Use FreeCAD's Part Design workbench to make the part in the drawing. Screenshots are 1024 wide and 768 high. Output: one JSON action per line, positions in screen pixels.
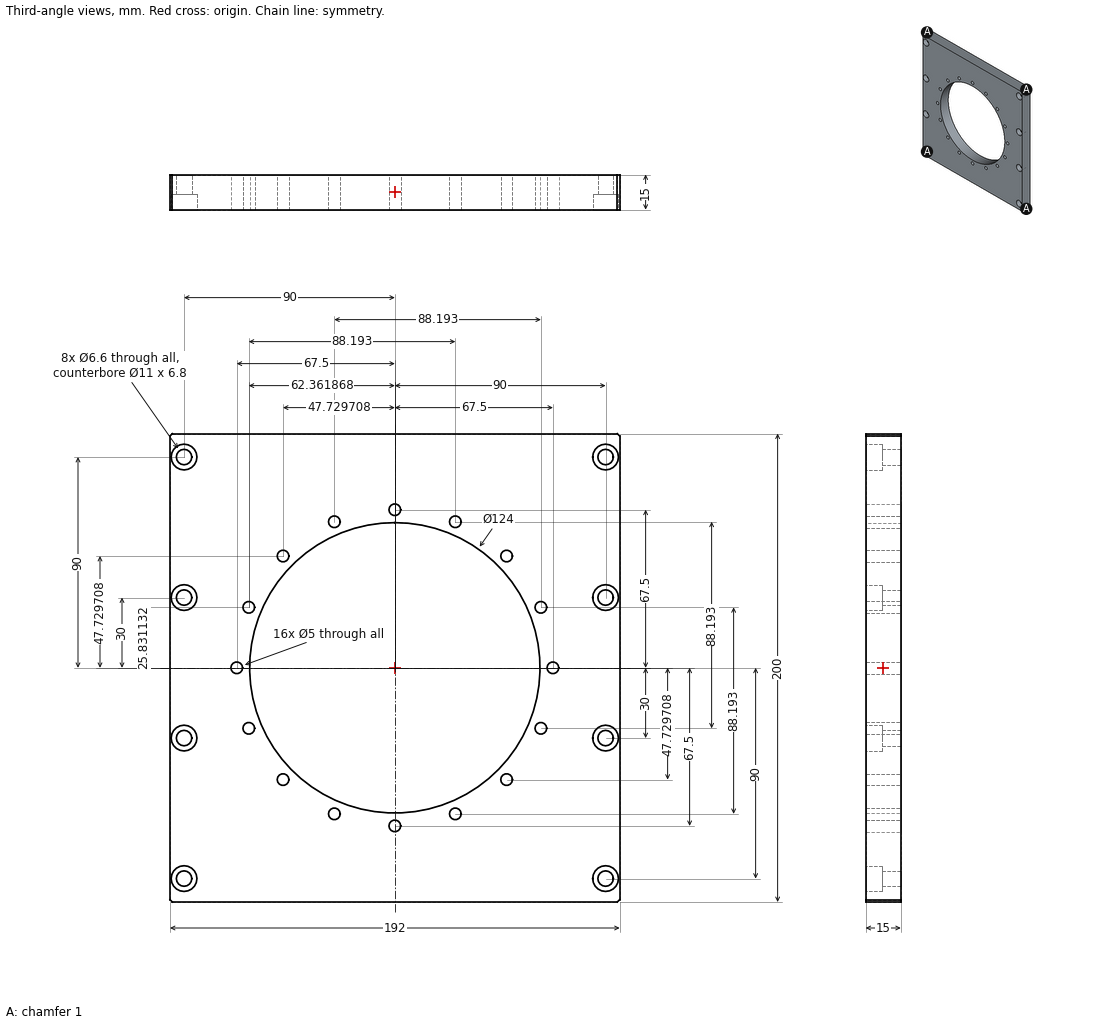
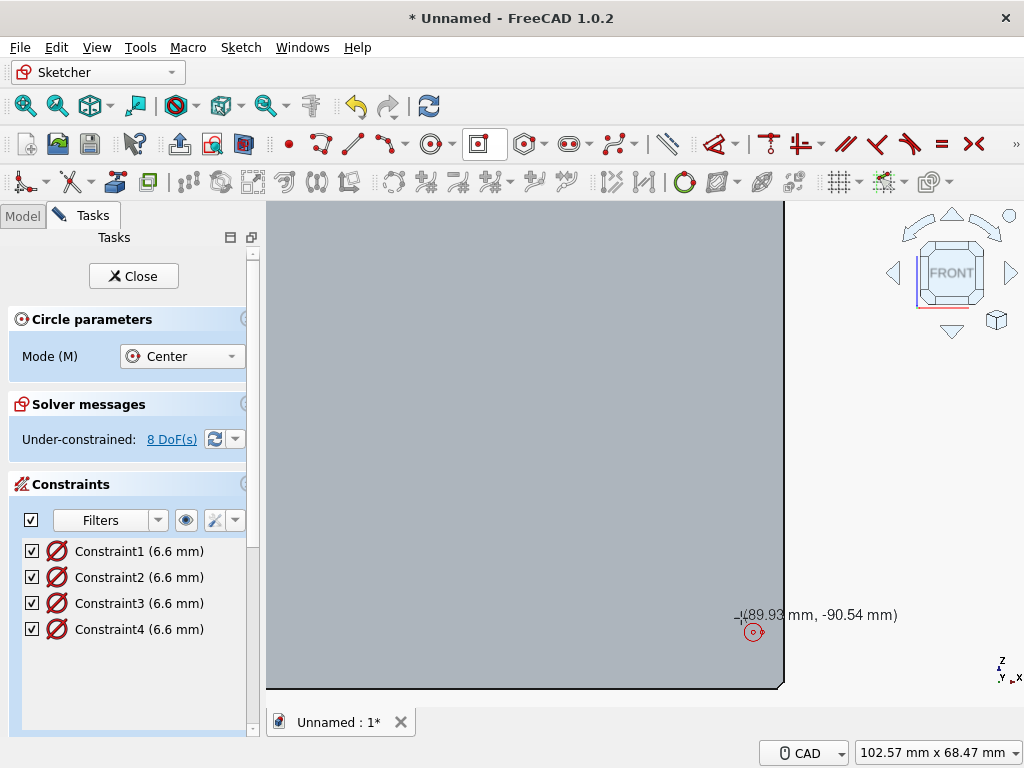
{"action": "scroll", "coordinate": [741, 619], "scroll_direction": "down", "scroll_amount": 7}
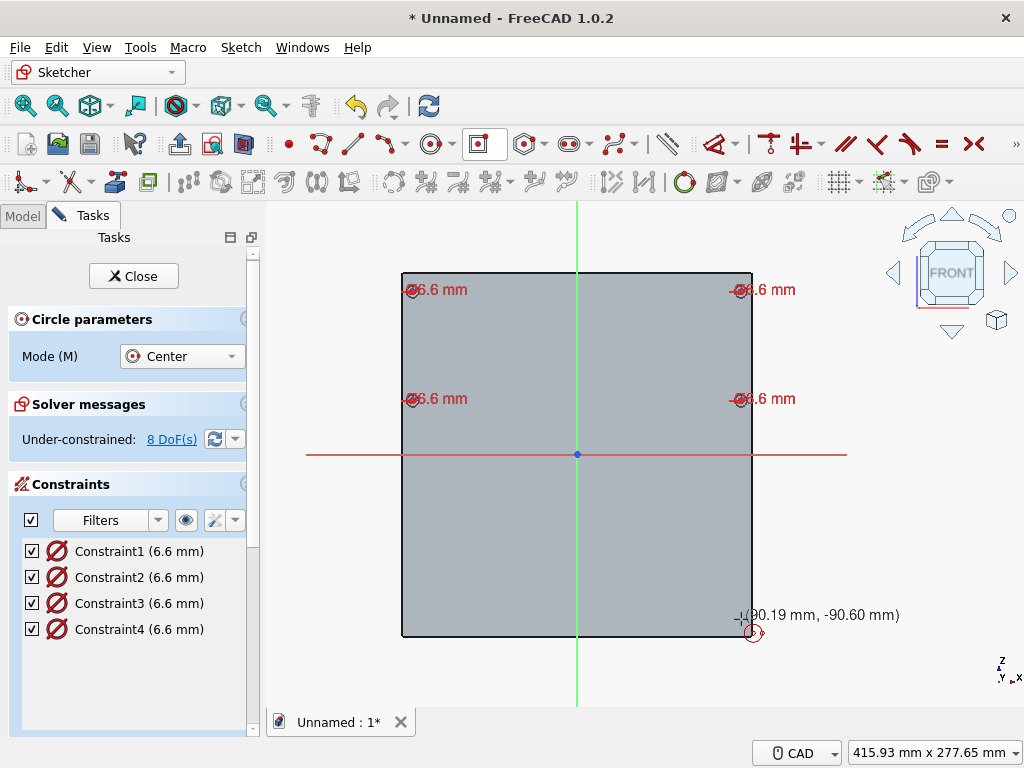
{"action": "left_click", "coordinate": [741, 619]}
{"action": "mouse_move", "coordinate": [745, 615]}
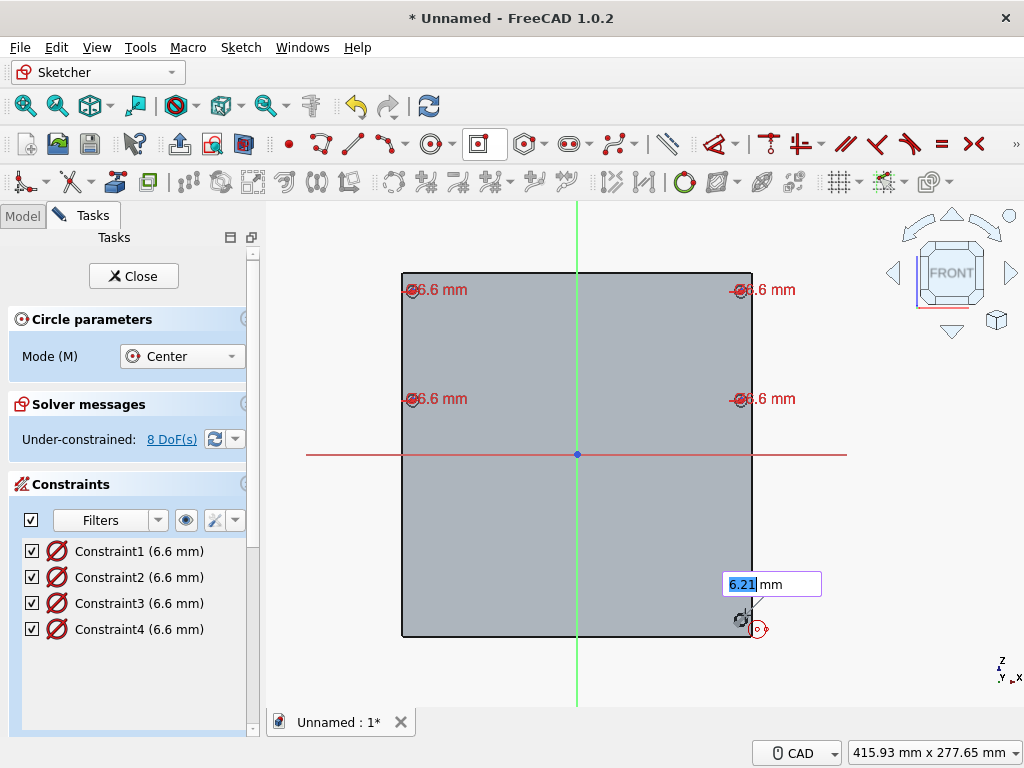
{"action": "type", "text": "6.6"}
{"action": "key", "text": "Return"}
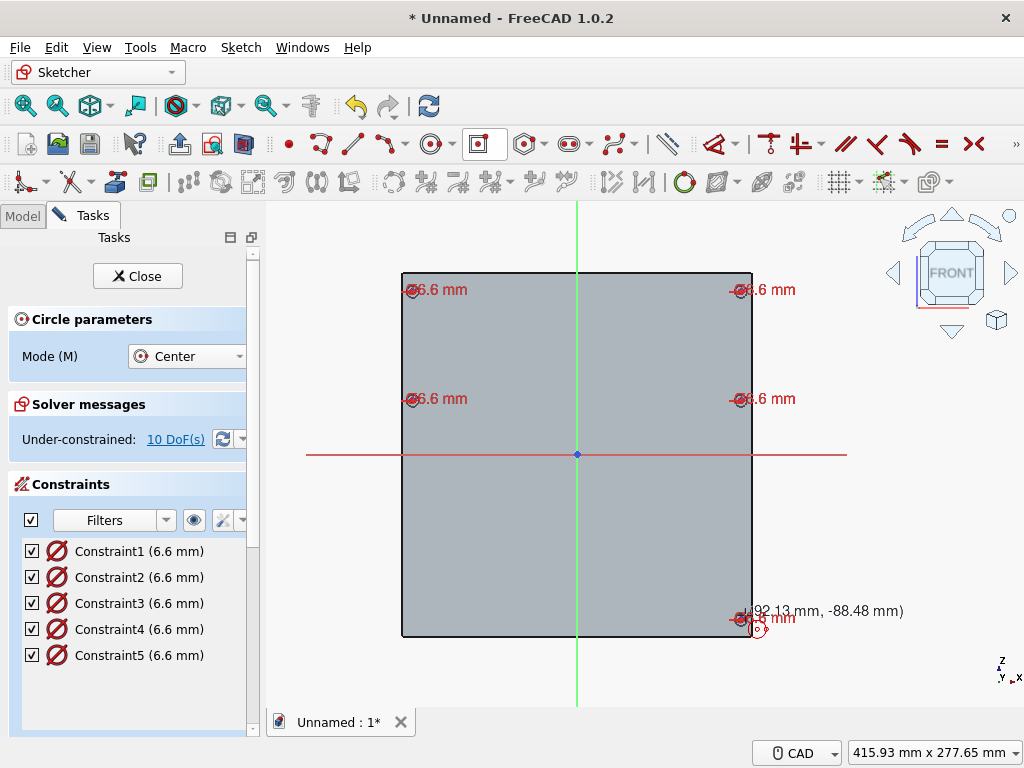
{"action": "scroll", "coordinate": [741, 509], "scroll_direction": "up", "scroll_amount": 7}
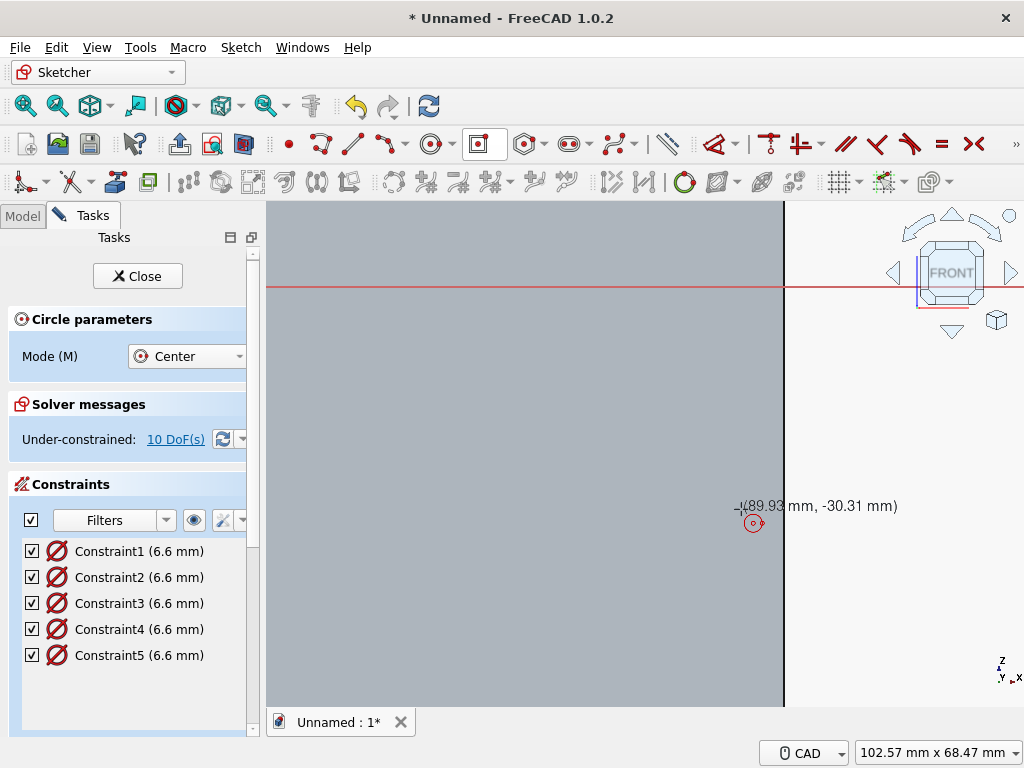
{"action": "scroll", "coordinate": [741, 509], "scroll_direction": "down", "scroll_amount": 7}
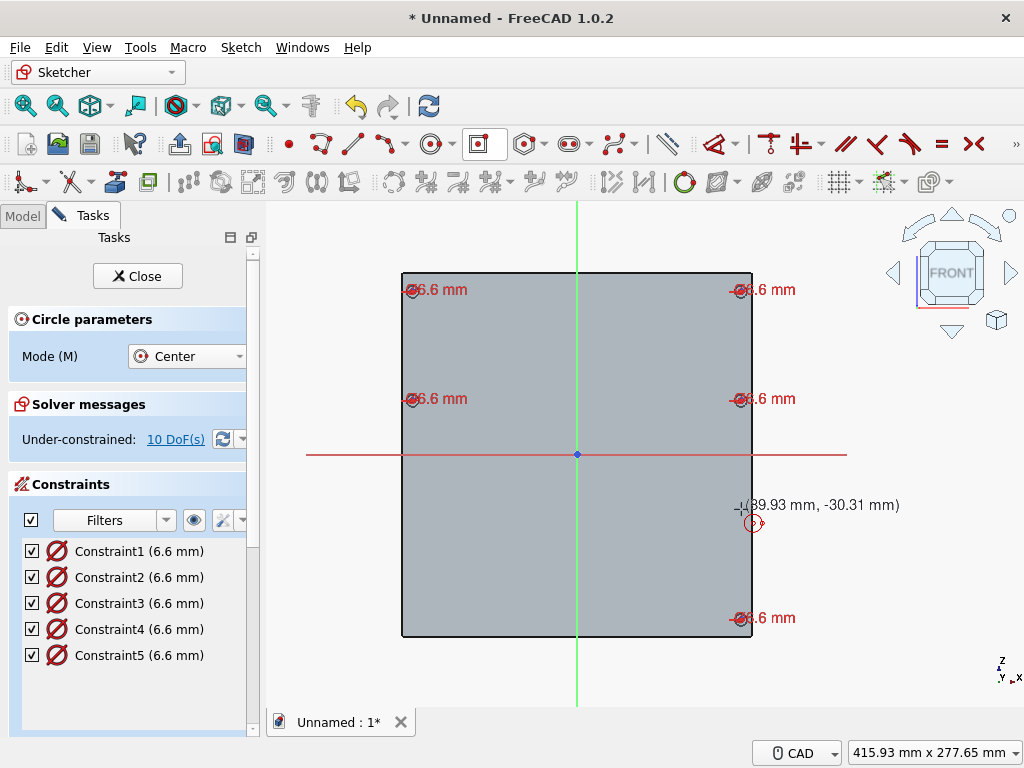
{"action": "left_click", "coordinate": [741, 509]}
{"action": "mouse_move", "coordinate": [745, 505]}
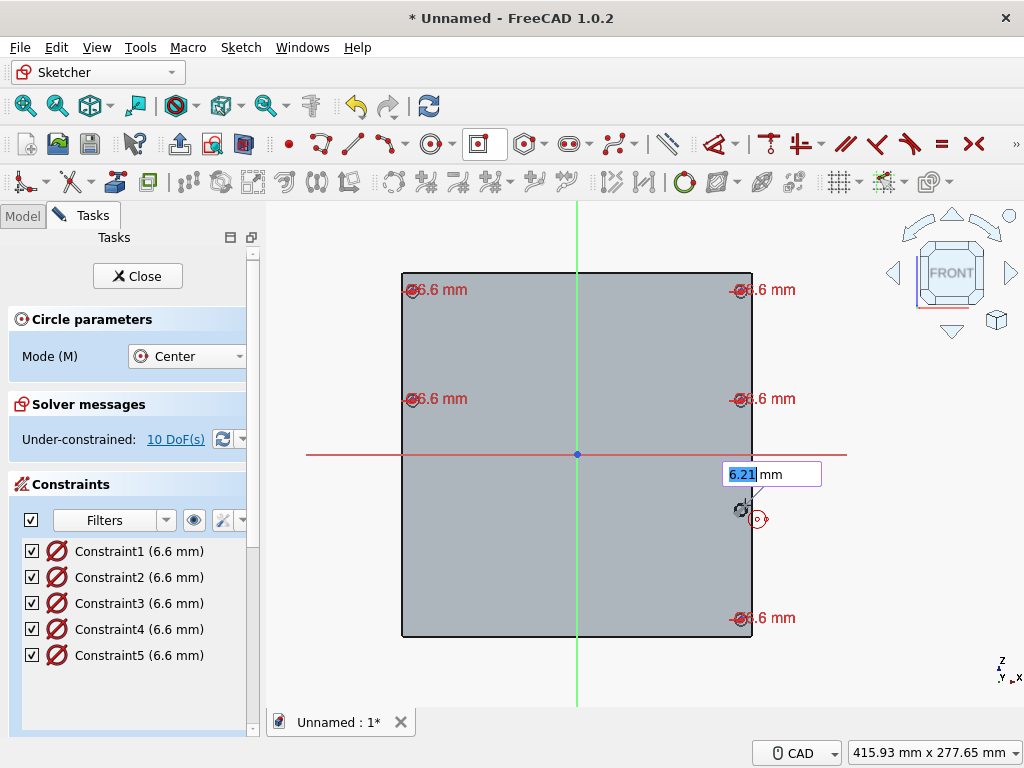
{"action": "type", "text": "6.6"}
{"action": "key", "text": "Return"}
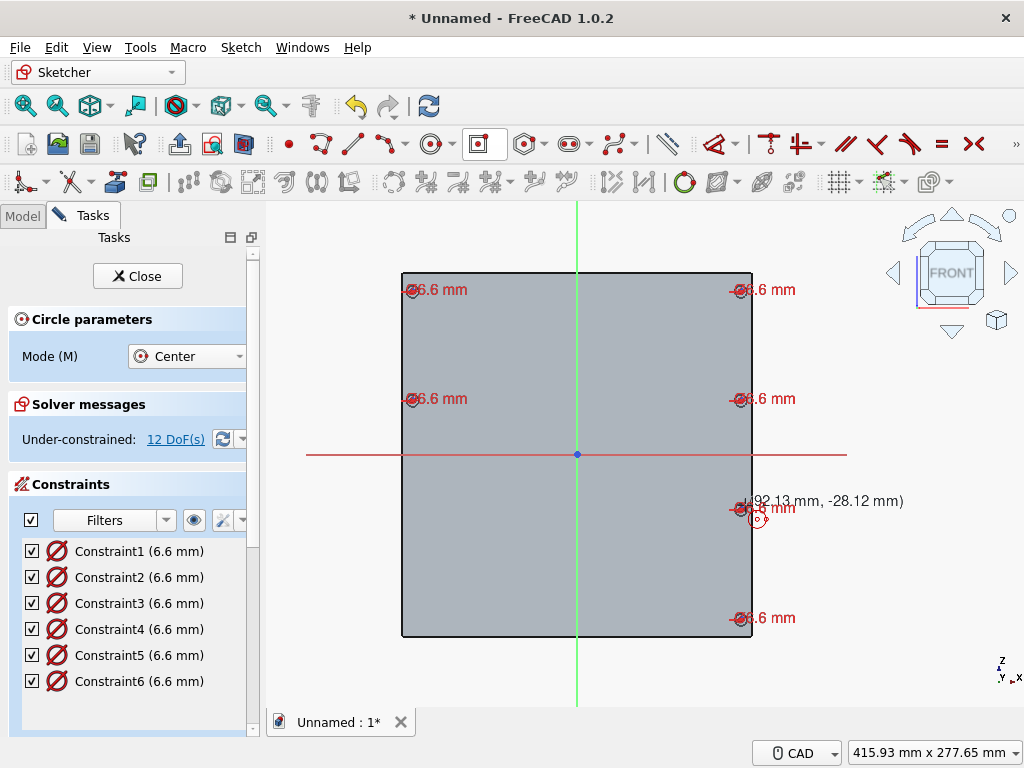
{"action": "scroll", "coordinate": [413, 509], "scroll_direction": "up", "scroll_amount": 7}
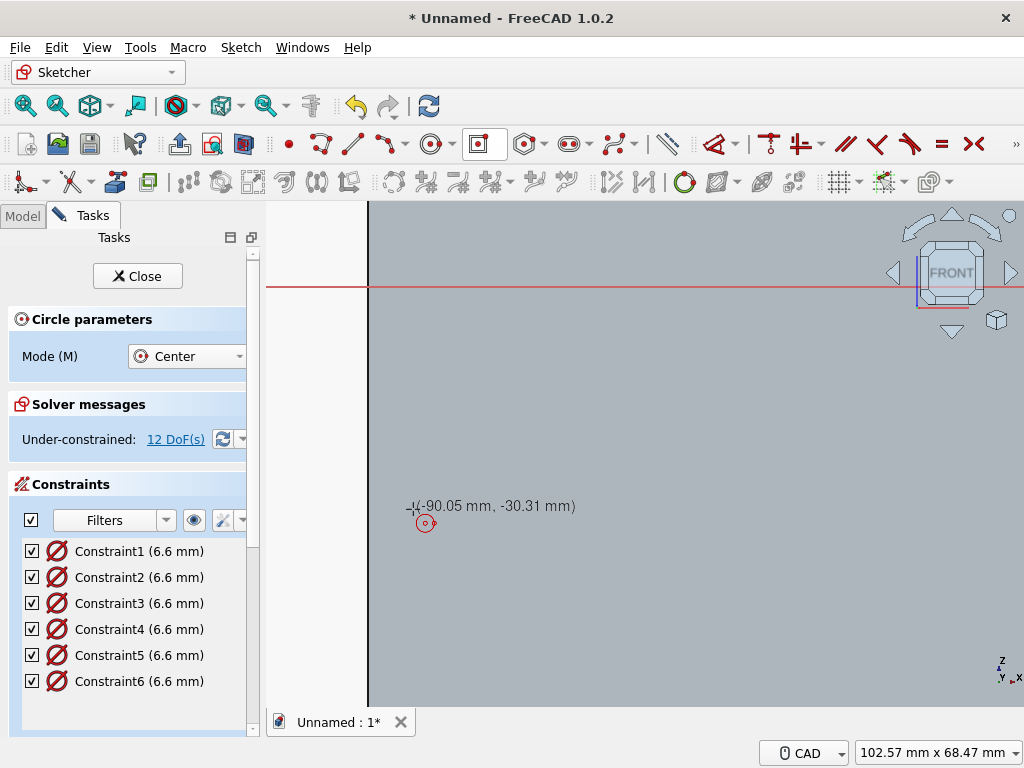
{"action": "scroll", "coordinate": [412, 509], "scroll_direction": "down", "scroll_amount": 7}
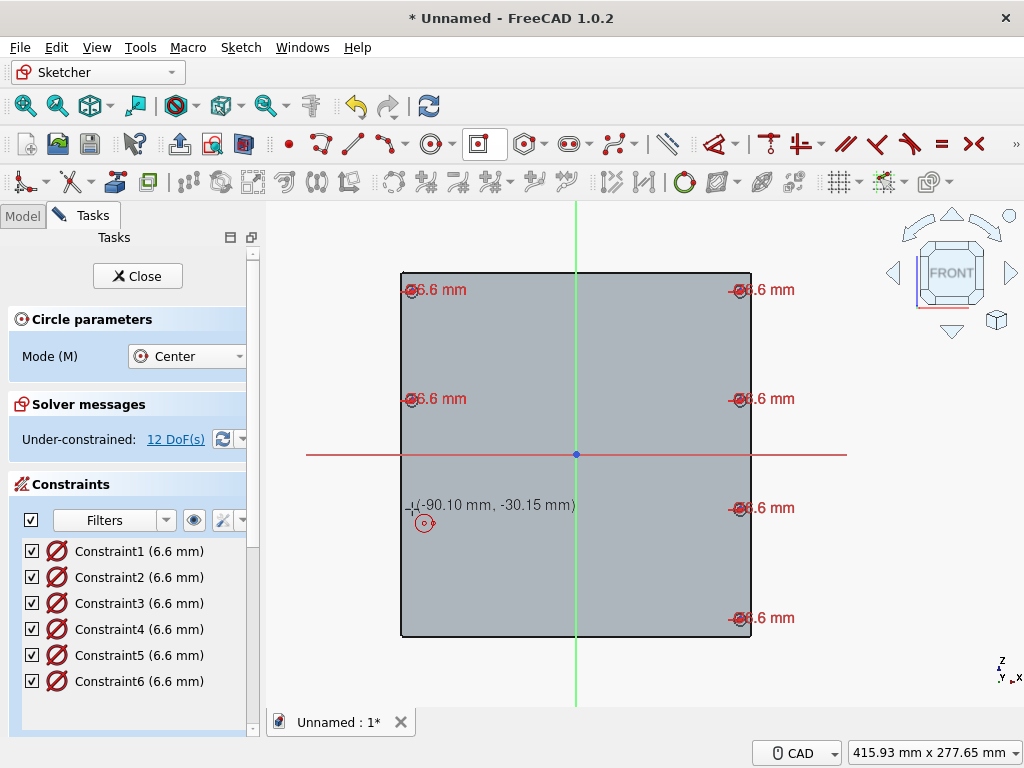
{"action": "left_click", "coordinate": [412, 509]}
{"action": "mouse_move", "coordinate": [417, 505]}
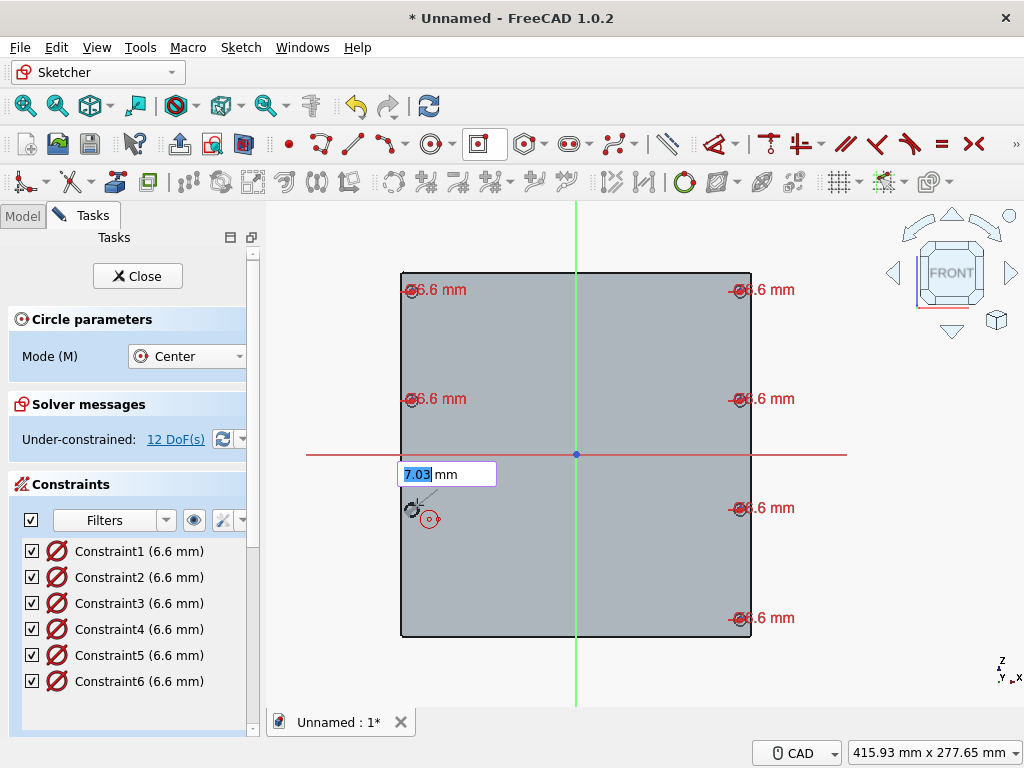
{"action": "type", "text": "6.6"}
{"action": "key", "text": "Return"}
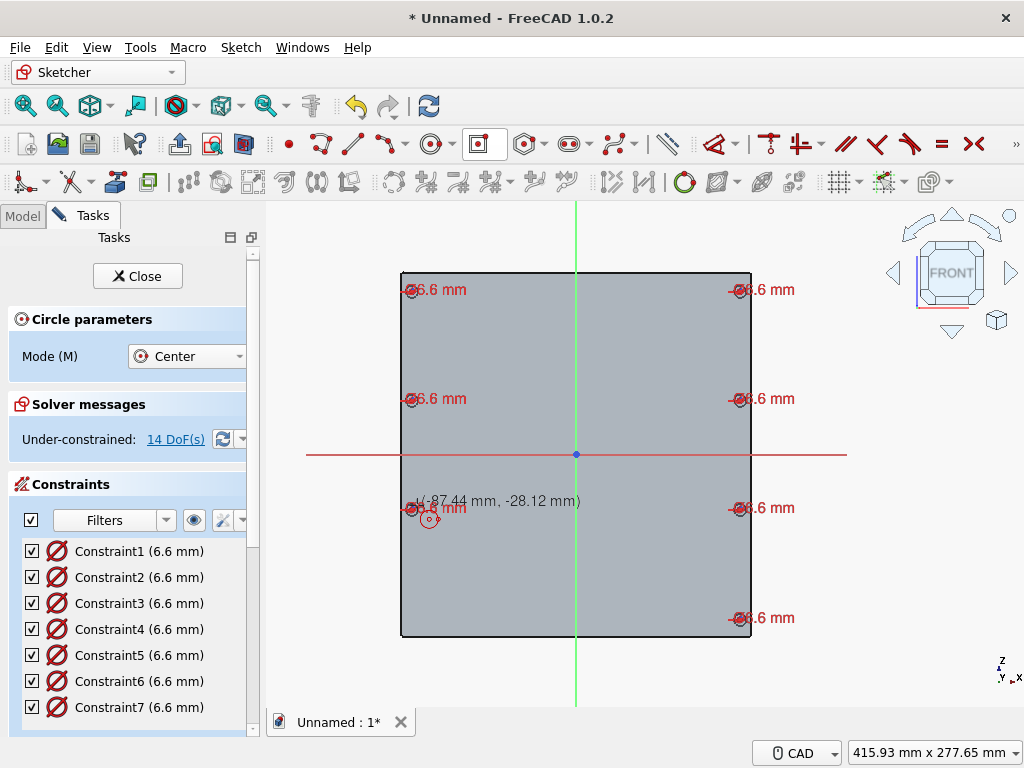
{"action": "scroll", "coordinate": [412, 619], "scroll_direction": "up", "scroll_amount": 7}